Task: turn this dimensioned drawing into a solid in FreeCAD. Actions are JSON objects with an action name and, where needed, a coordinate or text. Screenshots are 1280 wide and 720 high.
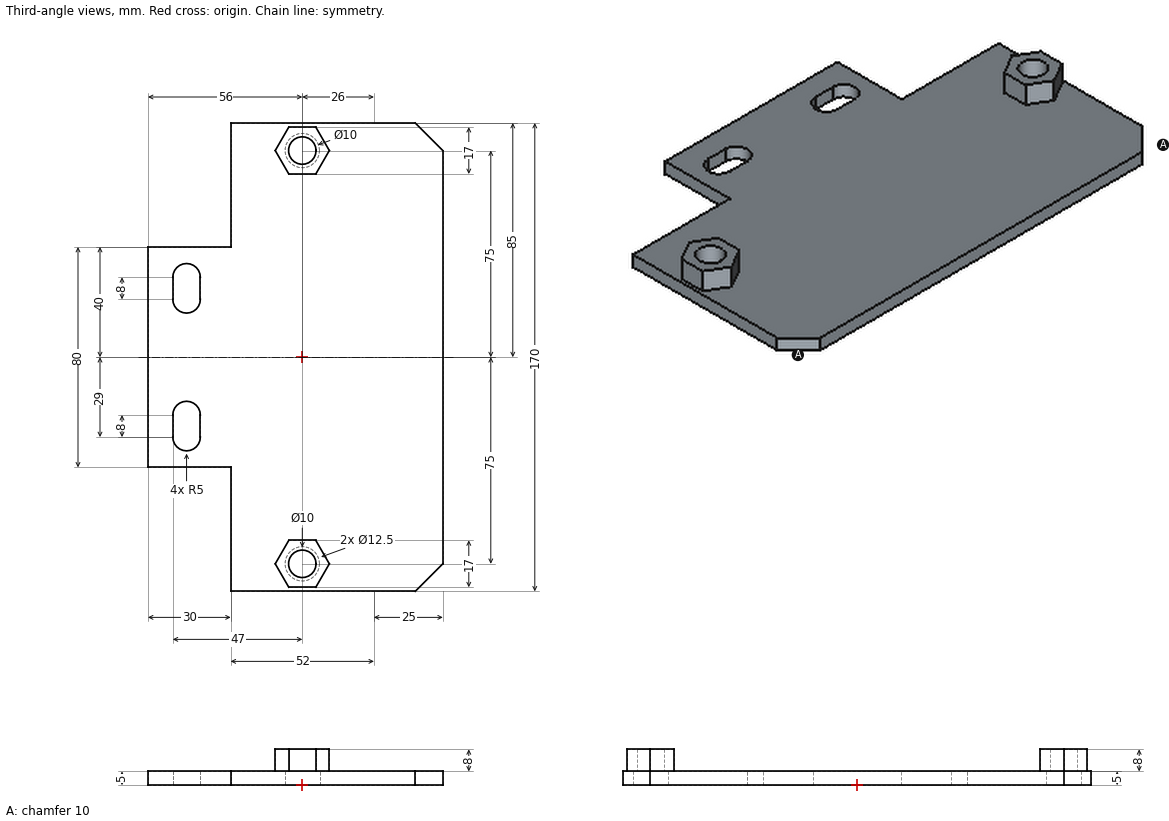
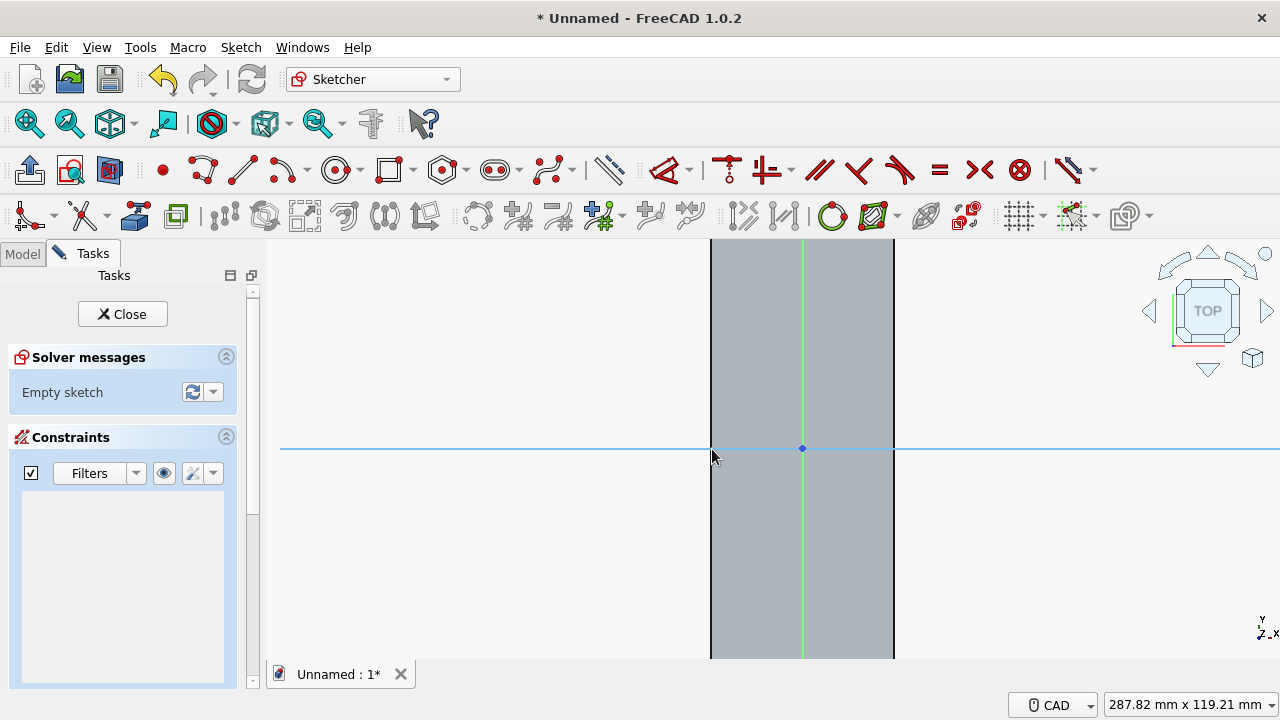
{"action": "left_click", "coordinate": [390, 170]}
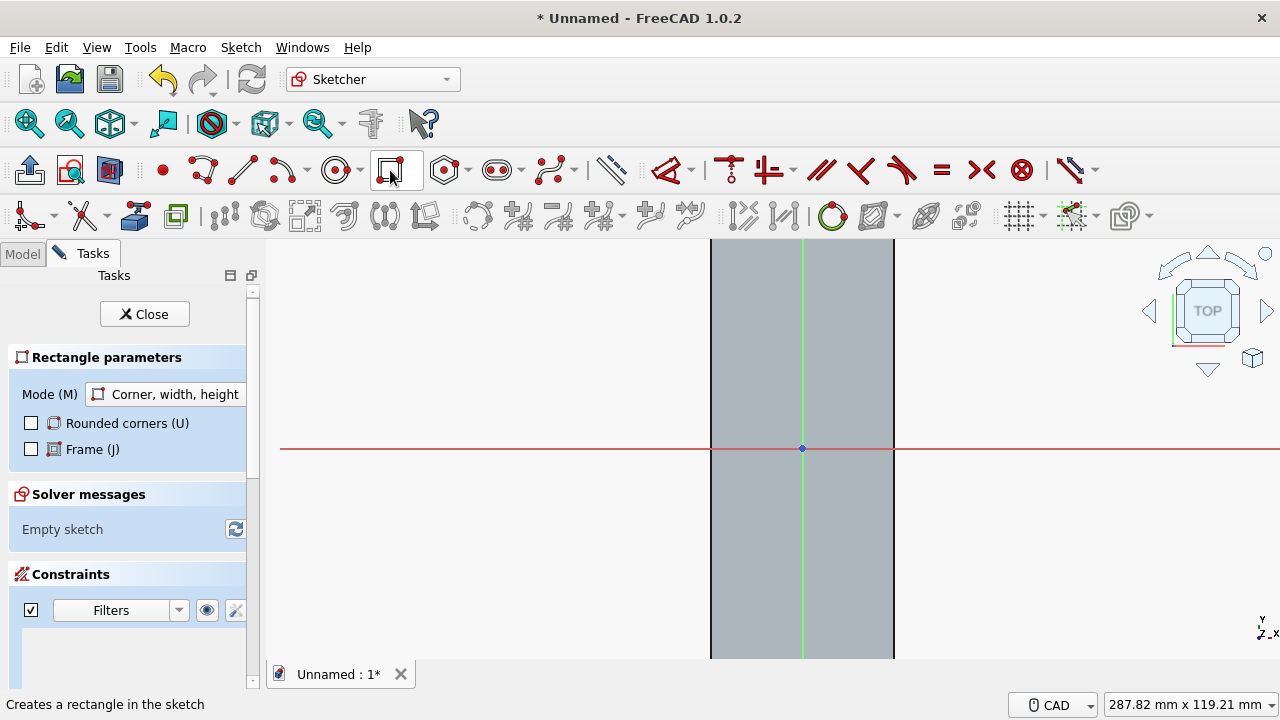
{"action": "left_click", "coordinate": [605, 308]}
{"action": "left_click", "coordinate": [711, 590]}
{"action": "key", "text": "Escape"}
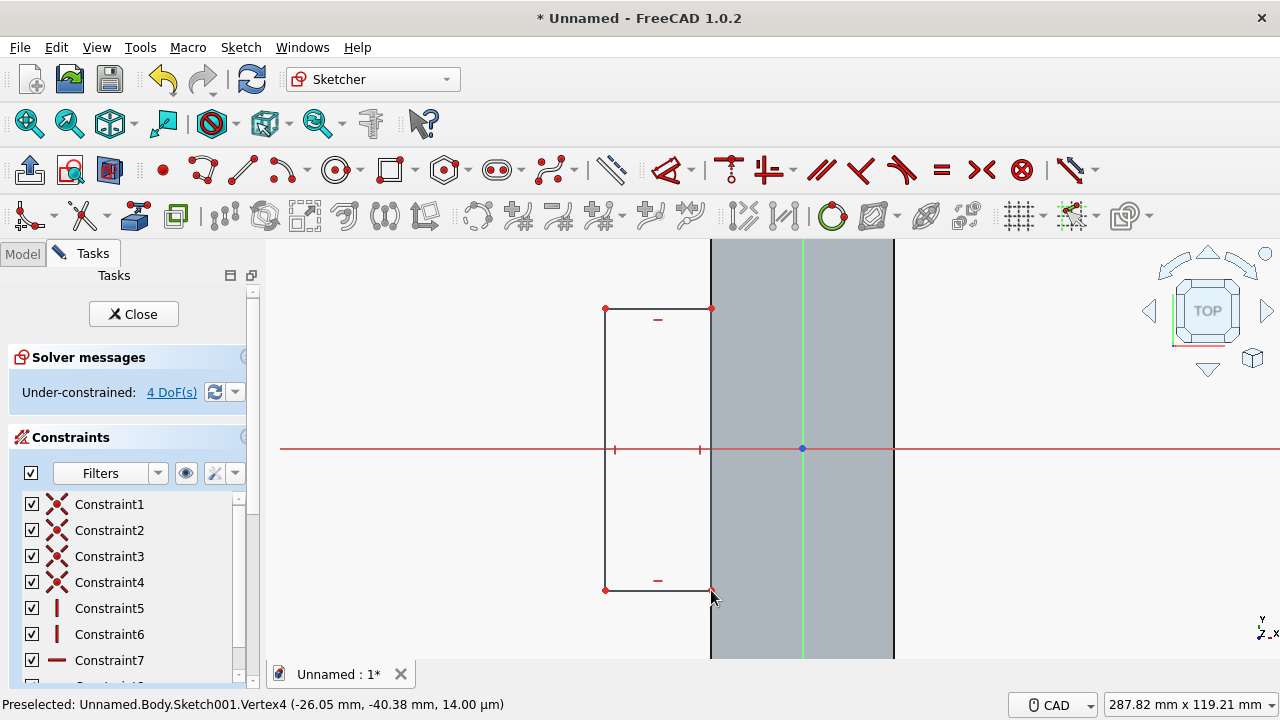
{"action": "left_click", "coordinate": [666, 170]}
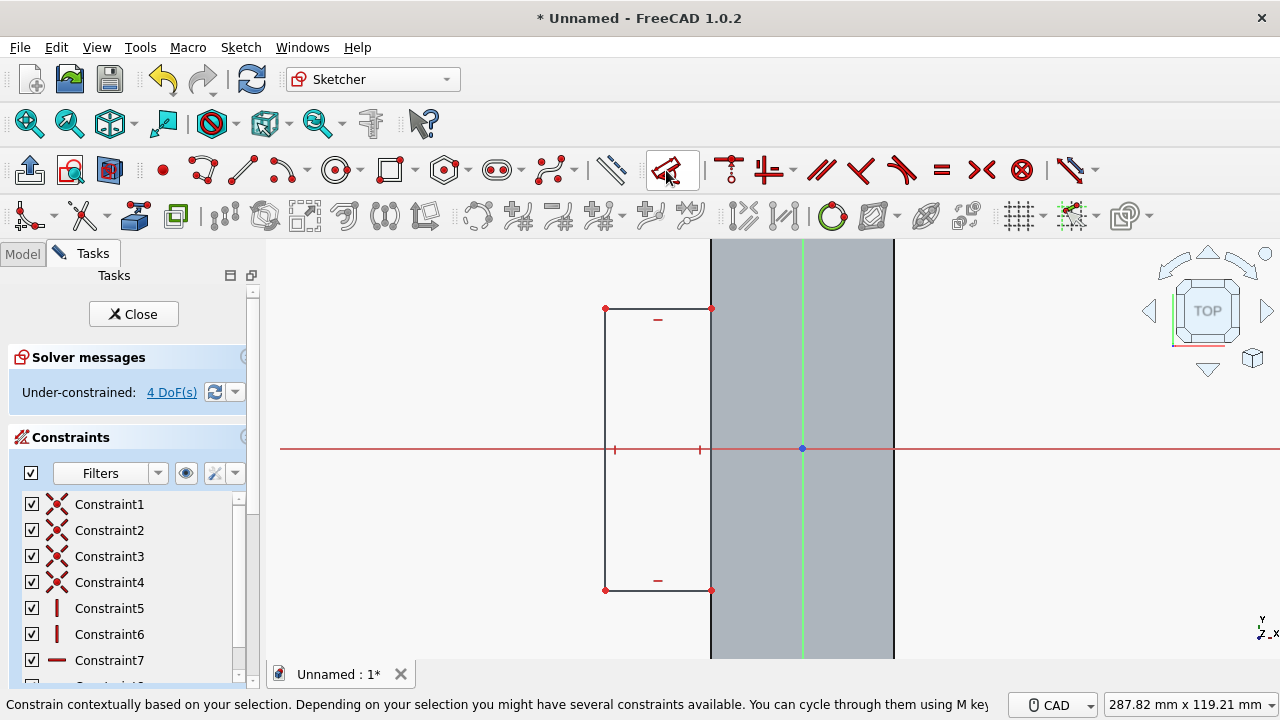
{"action": "left_click", "coordinate": [605, 394]}
{"action": "left_click", "coordinate": [571, 385]}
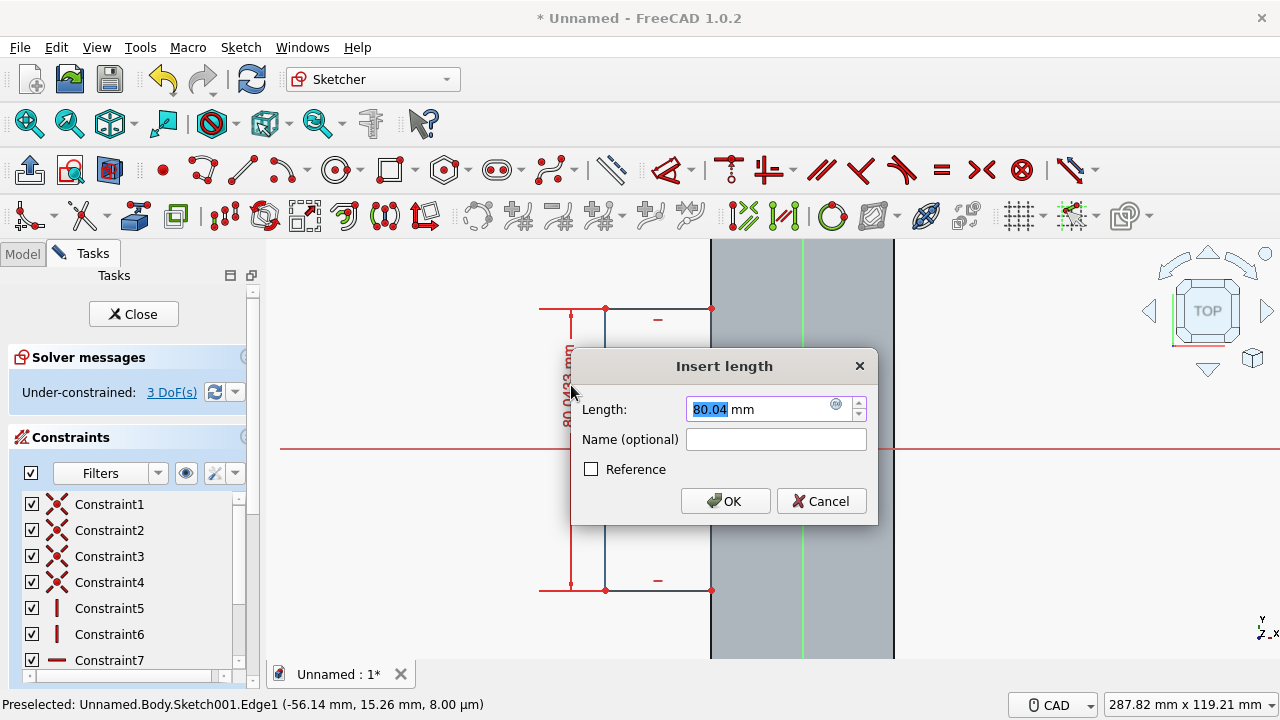
{"action": "type", "text": "80"}
{"action": "key", "text": "Return"}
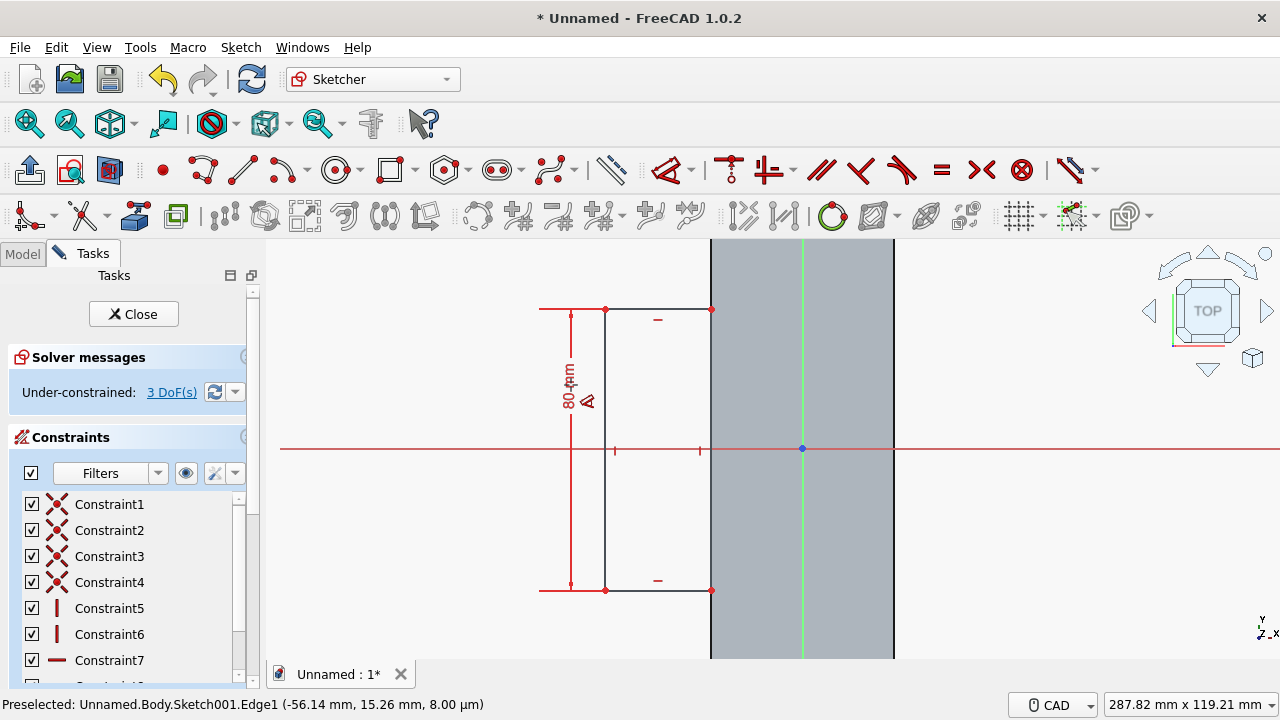
{"action": "left_click", "coordinate": [637, 591]}
{"action": "left_click", "coordinate": [658, 625]}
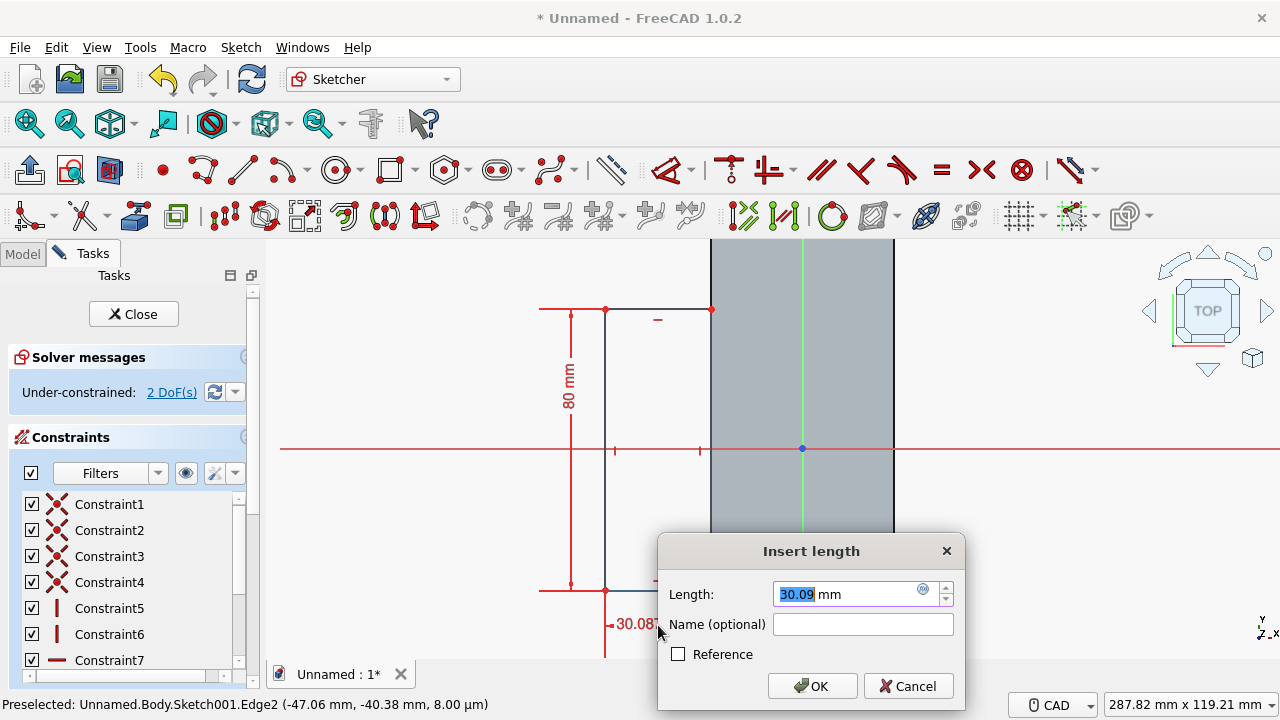
{"action": "type", "text": "30"}
{"action": "key", "text": "Return"}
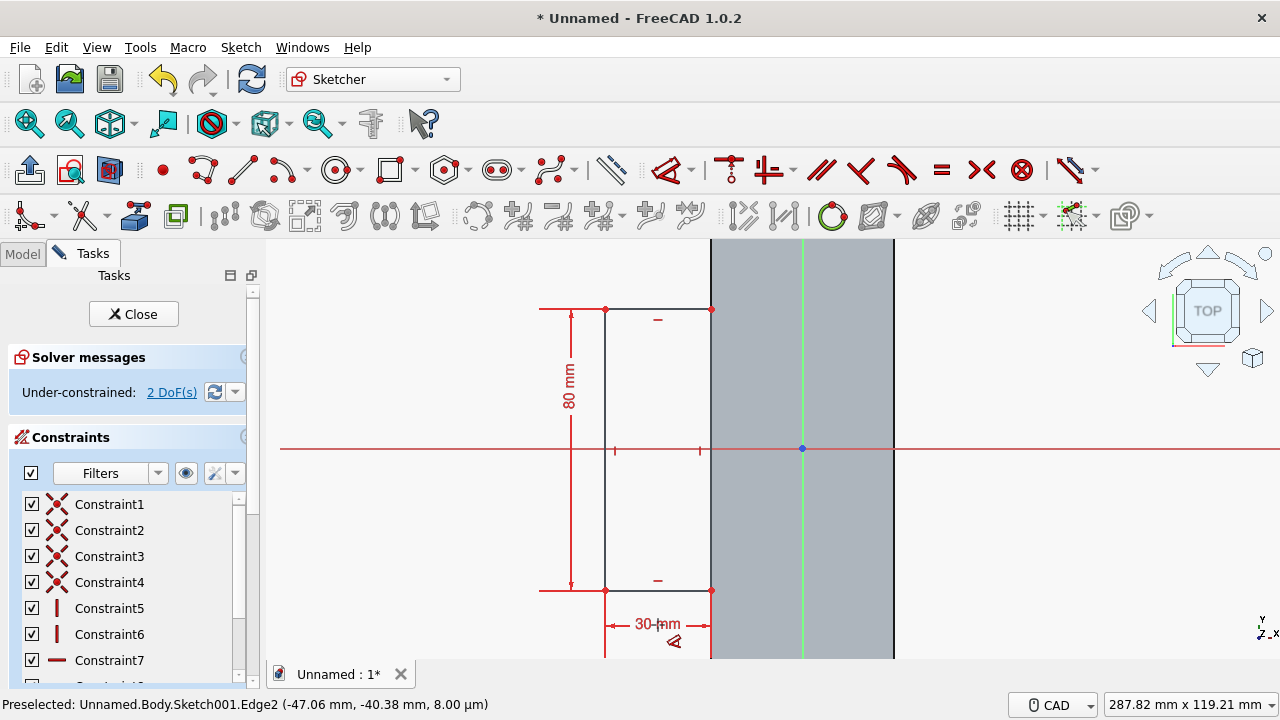
{"action": "left_click", "coordinate": [605, 309]}
{"action": "left_click", "coordinate": [704, 275]}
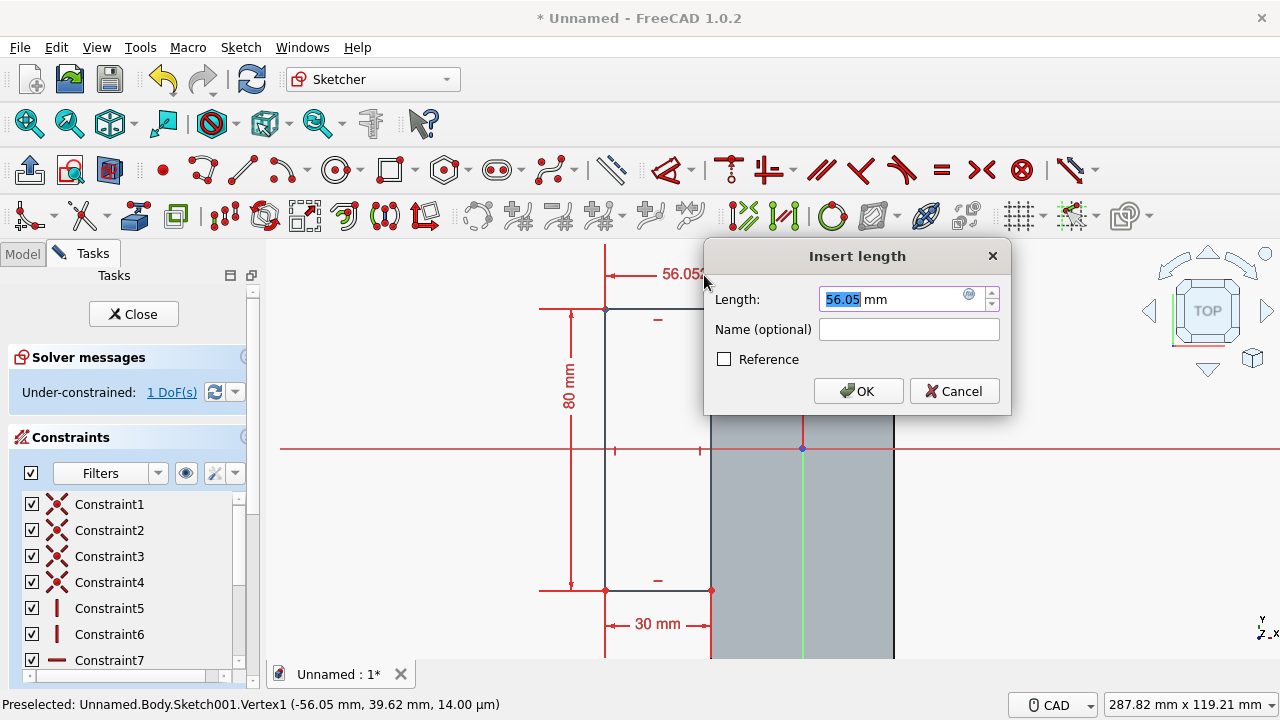
{"action": "type", "text": "56"}
{"action": "key", "text": "Return"}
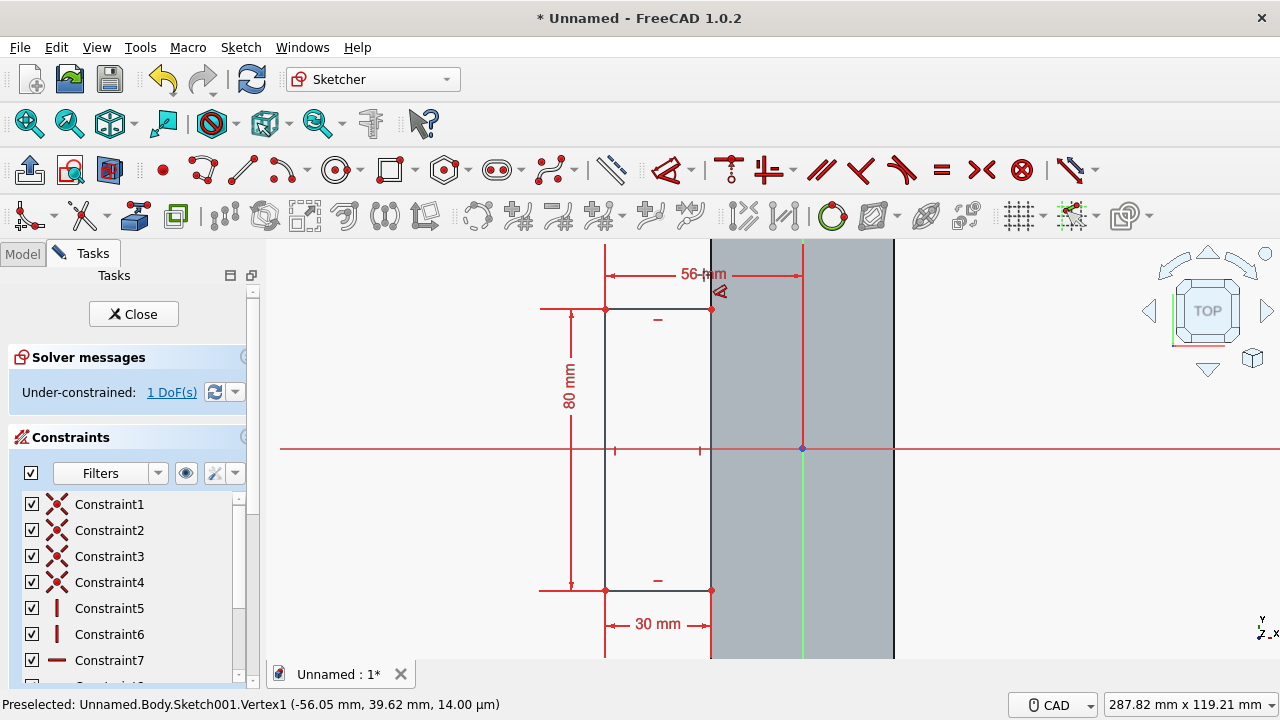
{"action": "left_click", "coordinate": [605, 309]}
{"action": "left_click", "coordinate": [571, 347]}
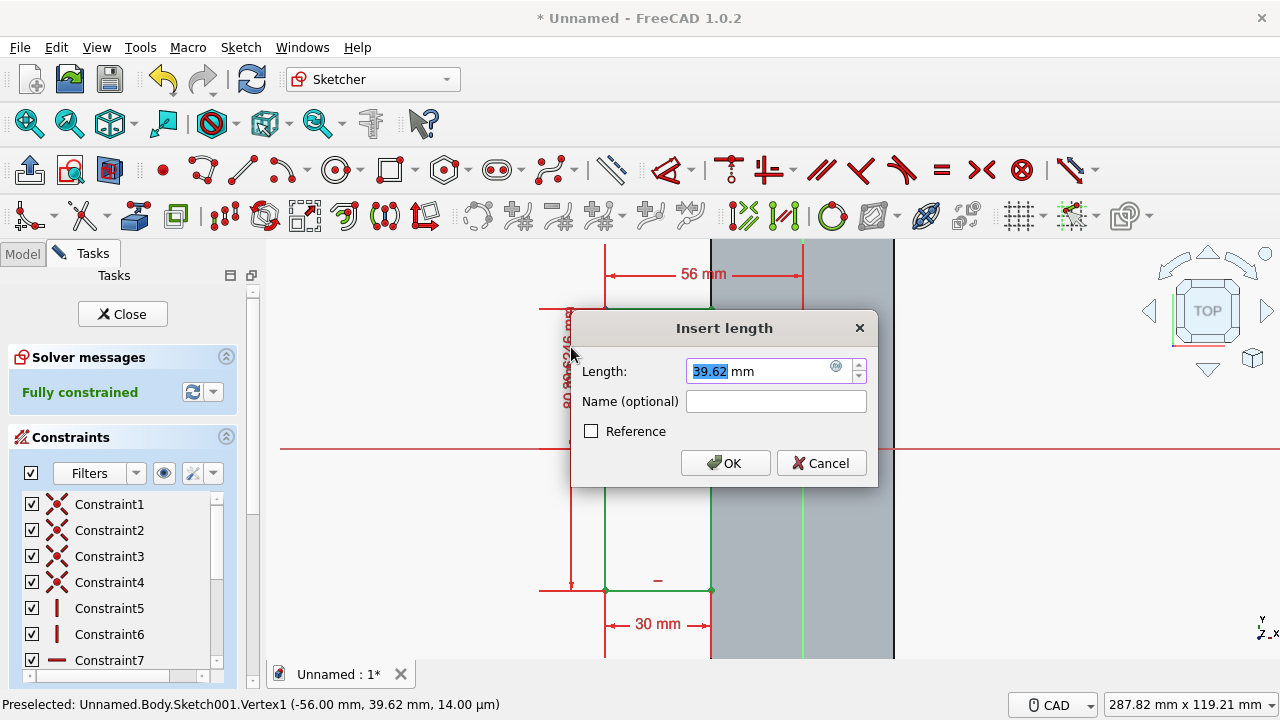
{"action": "type", "text": "40"}
{"action": "key", "text": "Return"}
{"action": "key", "text": "Escape"}